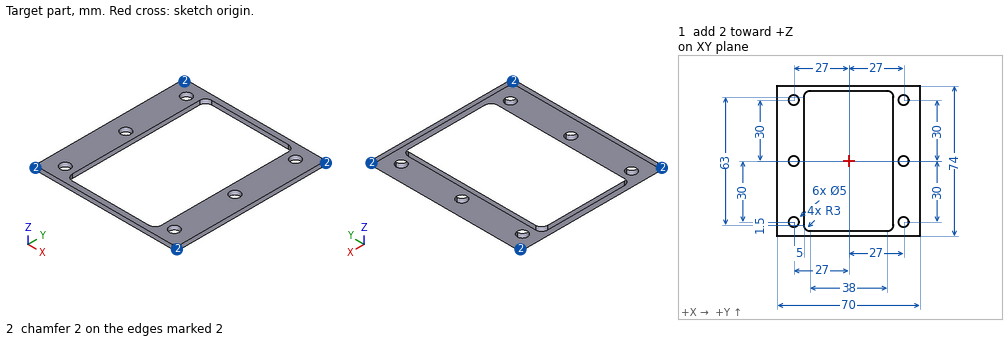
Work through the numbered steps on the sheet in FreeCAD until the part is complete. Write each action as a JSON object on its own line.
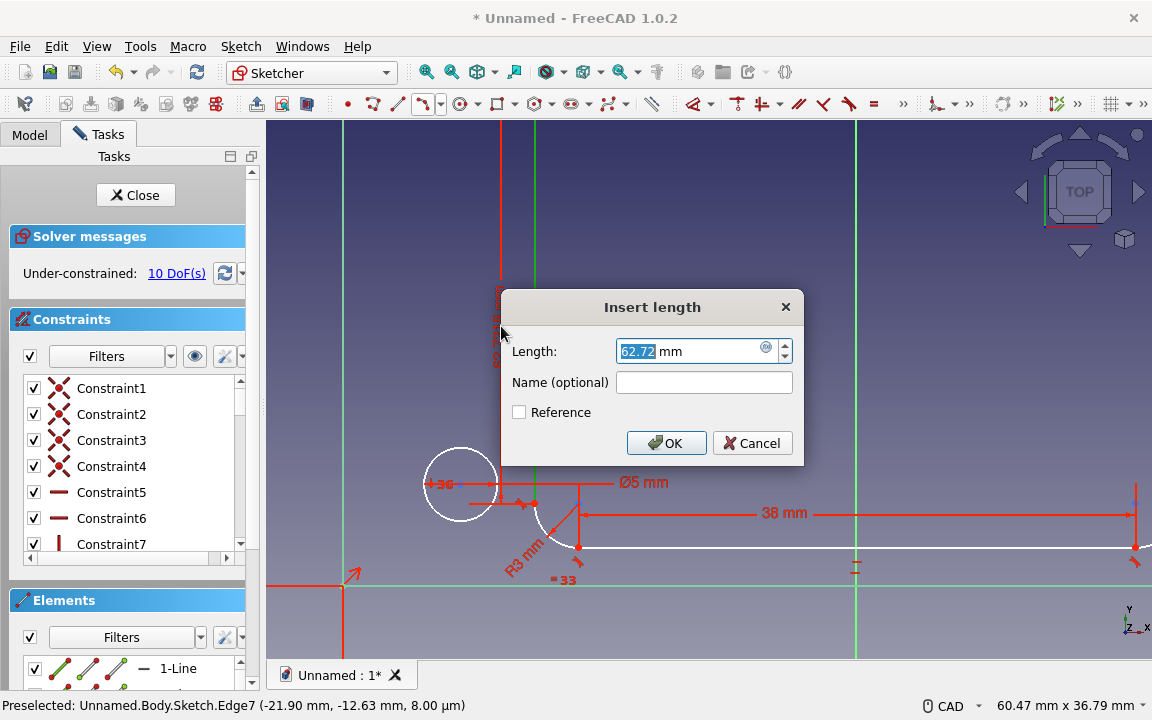
{"action": "type", "text": "63"}
{"action": "key", "text": "Return"}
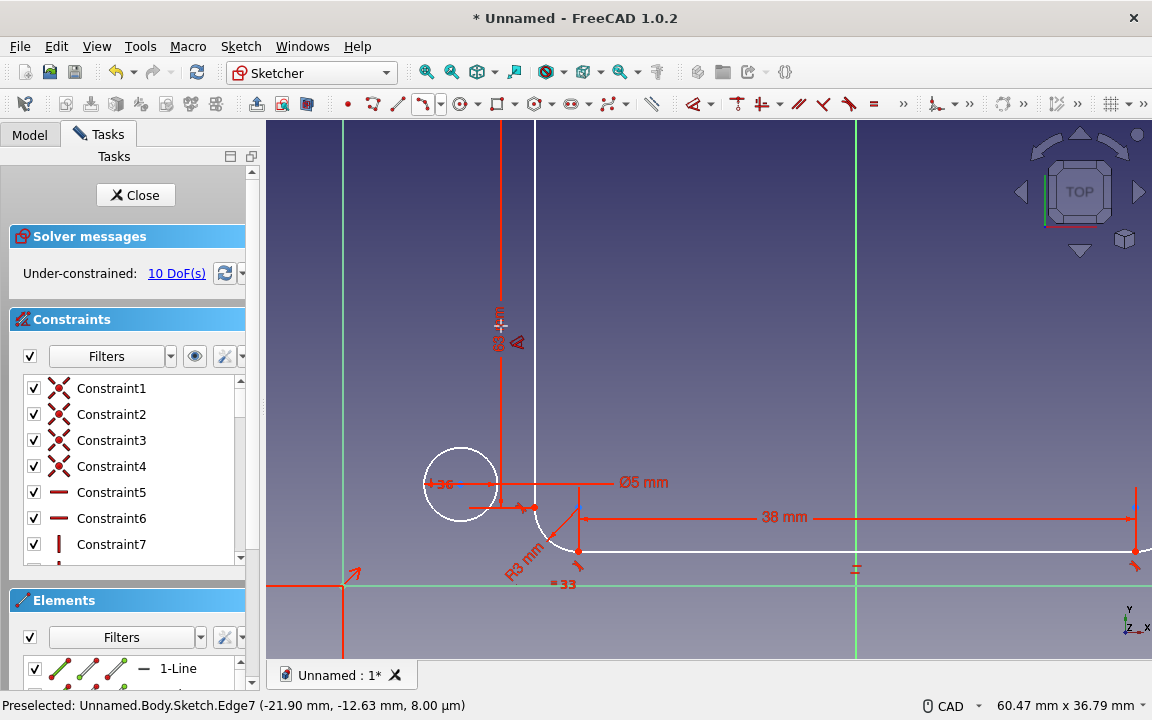
{"action": "left_click", "coordinate": [461, 484]}
{"action": "left_click", "coordinate": [658, 518]}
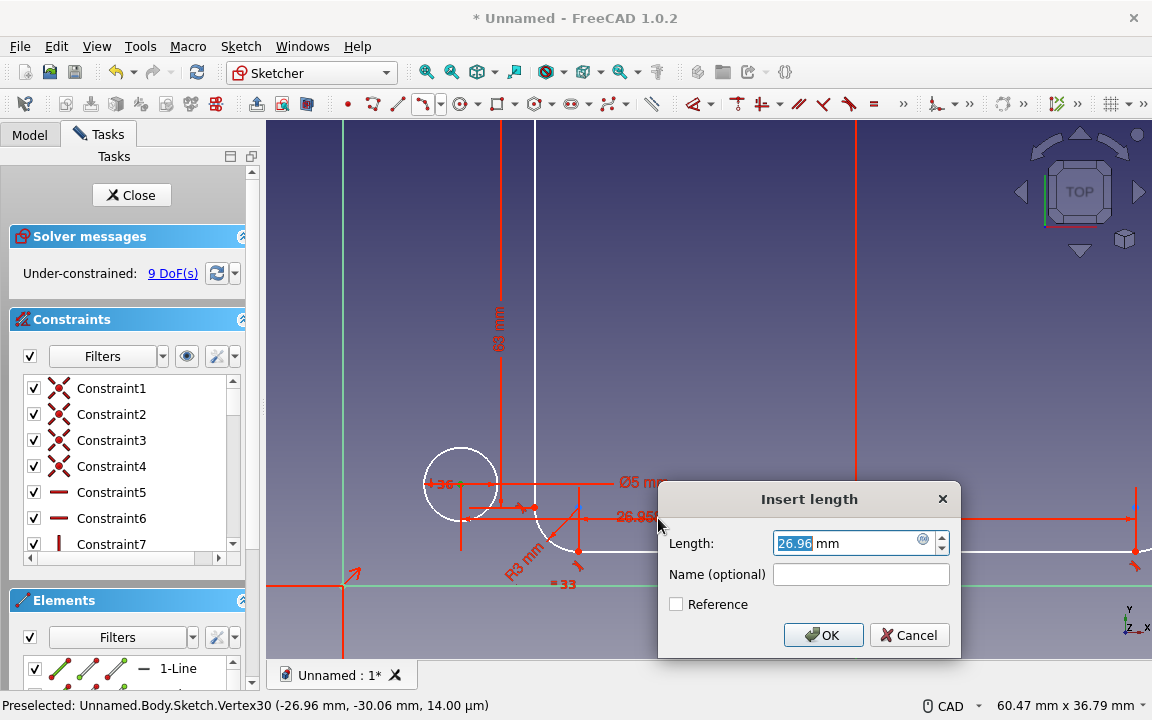
{"action": "type", "text": "27"}
{"action": "key", "text": "Return"}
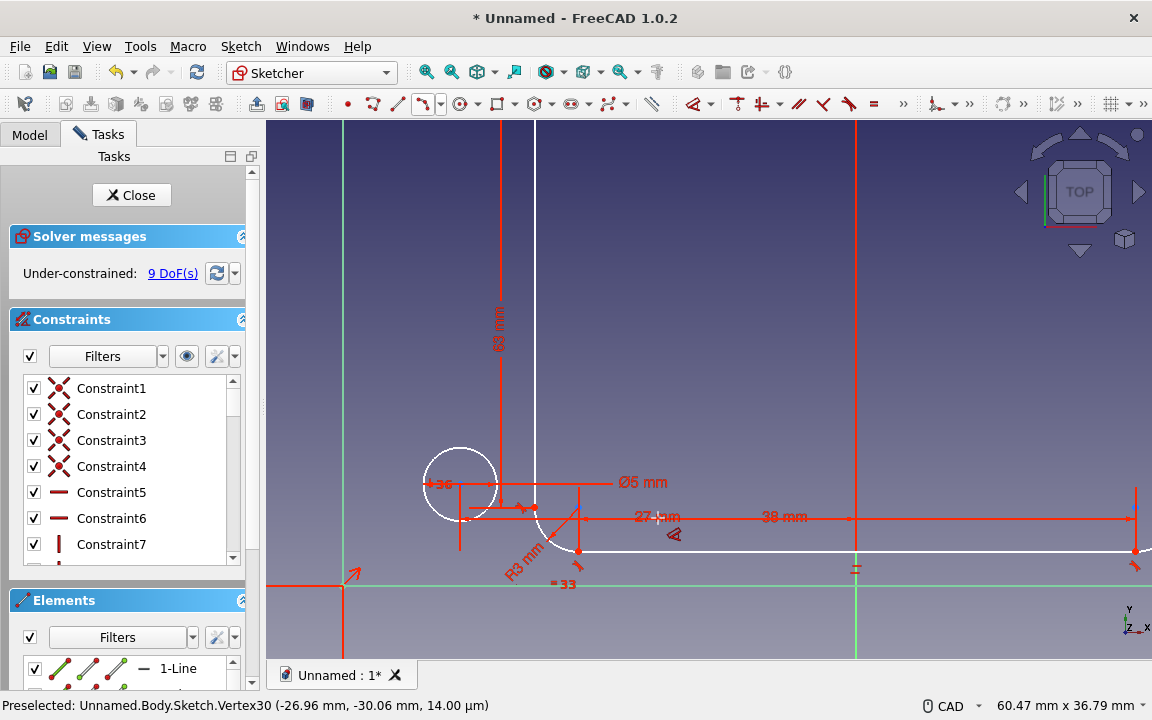
{"action": "left_click", "coordinate": [460, 484]}
{"action": "left_click", "coordinate": [426, 316]}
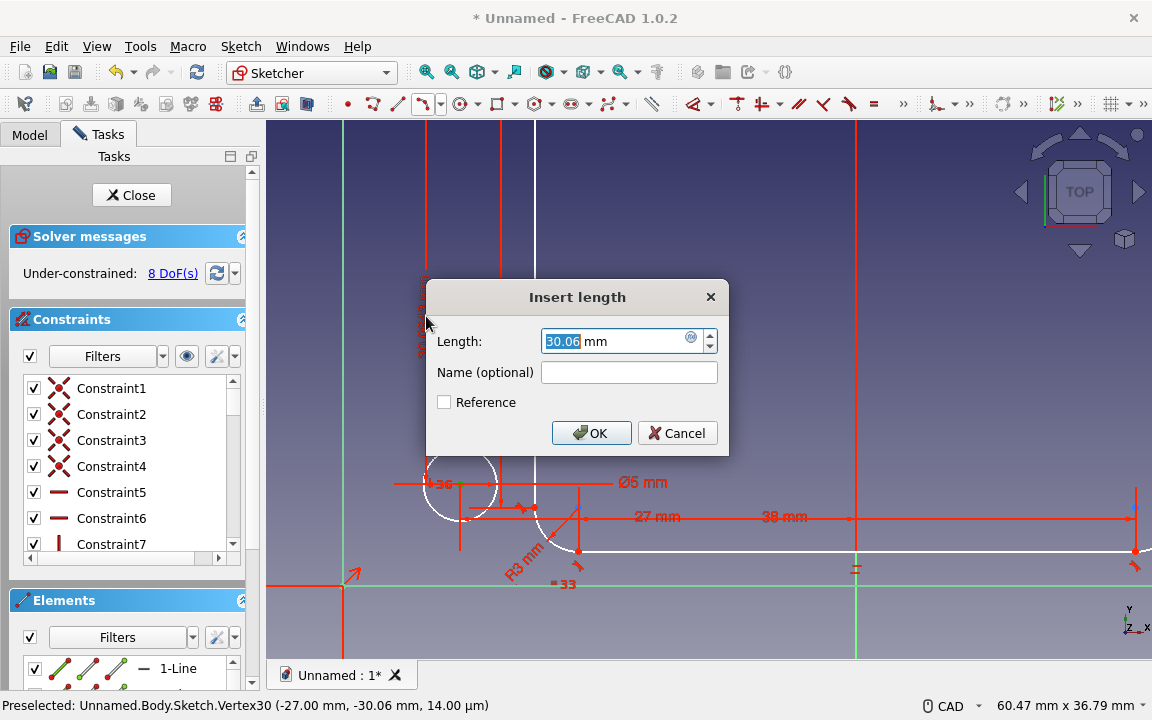
{"action": "type", "text": "30"}
{"action": "key", "text": "Return"}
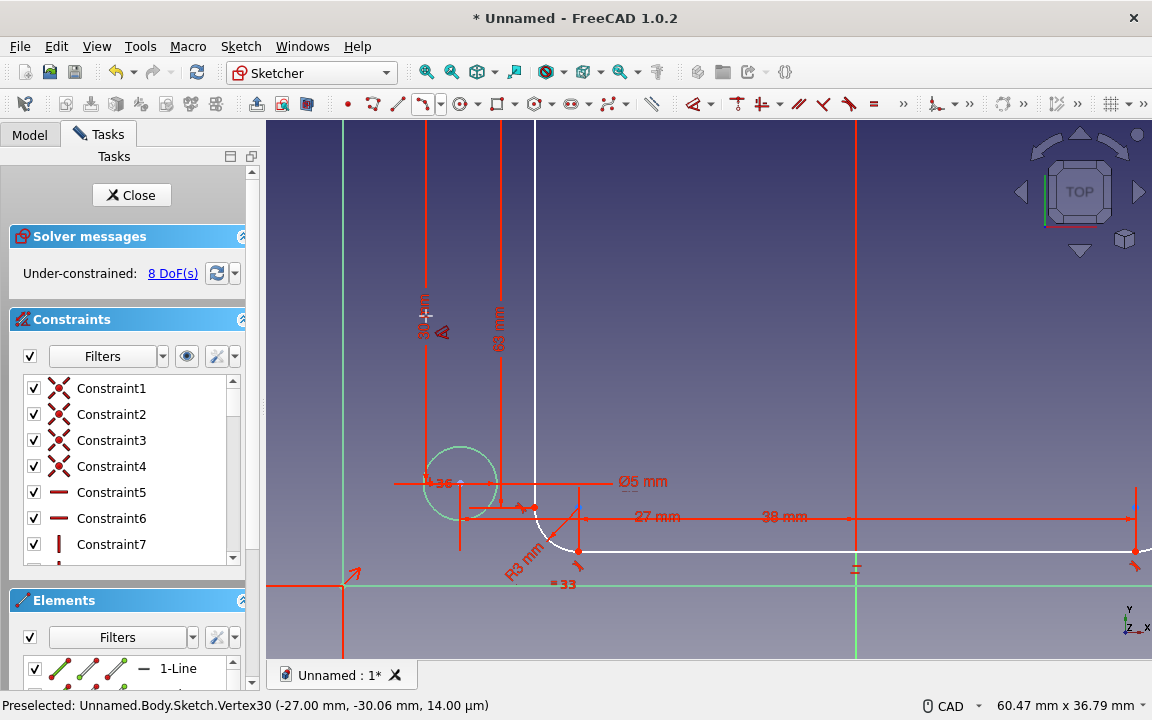
{"action": "scroll", "coordinate": [548, 538], "scroll_direction": "down", "scroll_amount": 6}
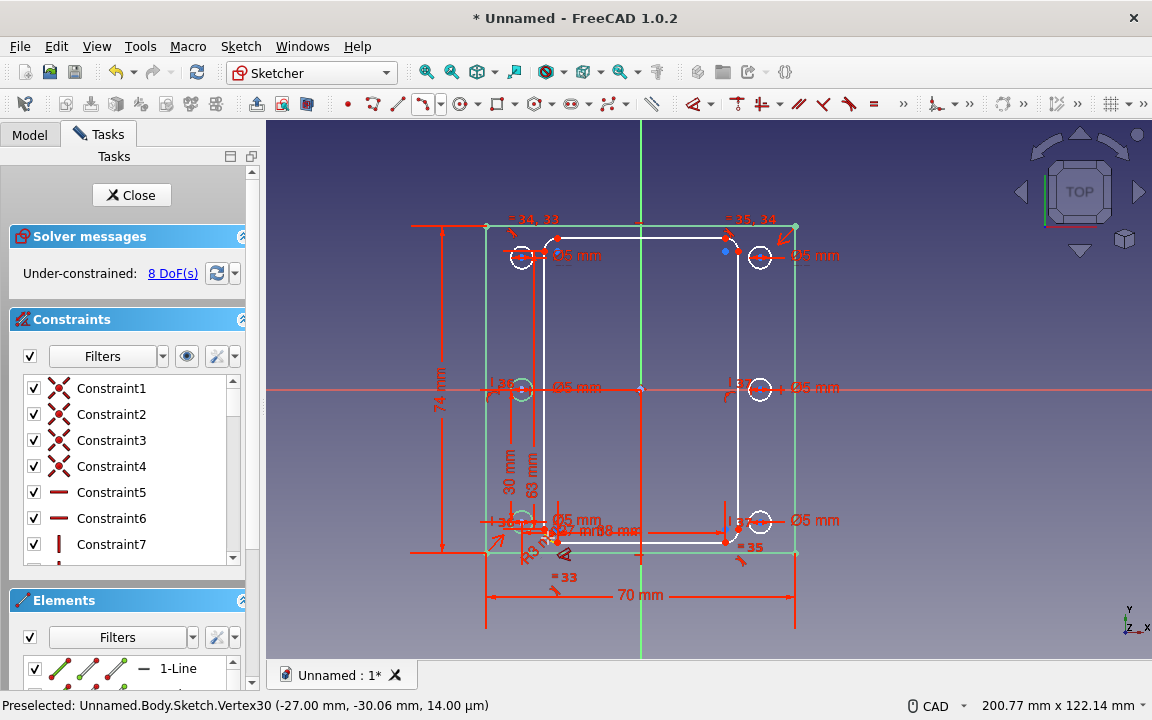
{"action": "left_click", "coordinate": [760, 522]}
{"action": "left_click", "coordinate": [701, 356]}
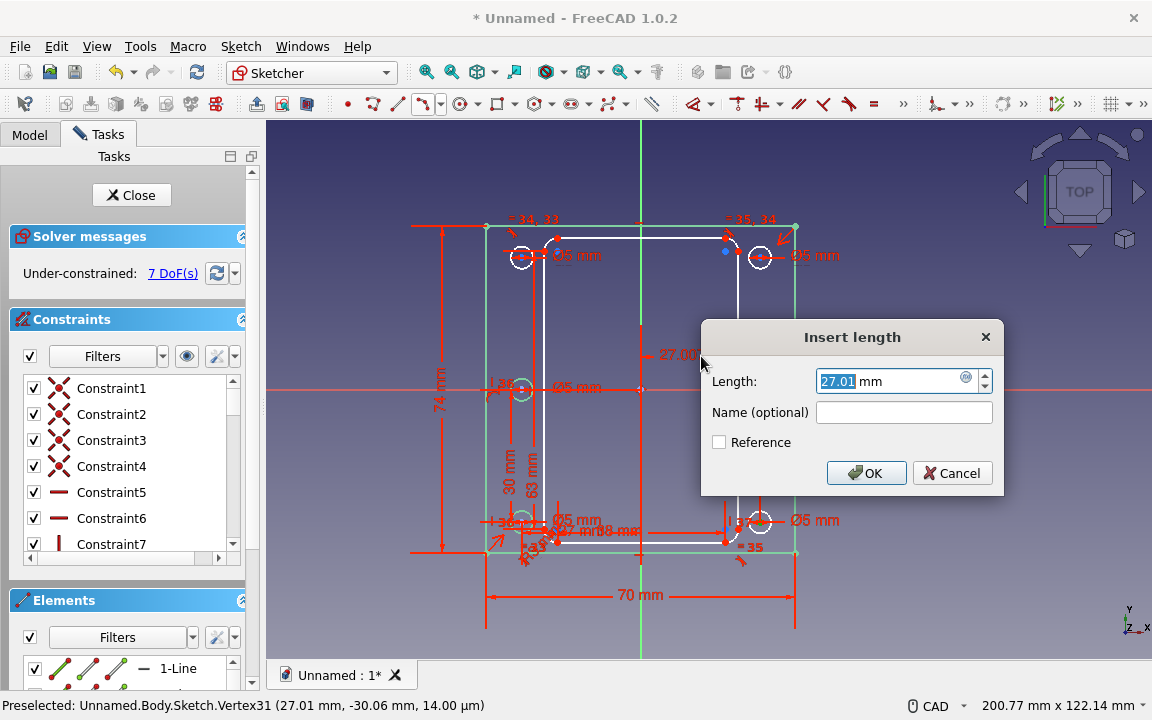
{"action": "type", "text": "27"}
{"action": "key", "text": "Return"}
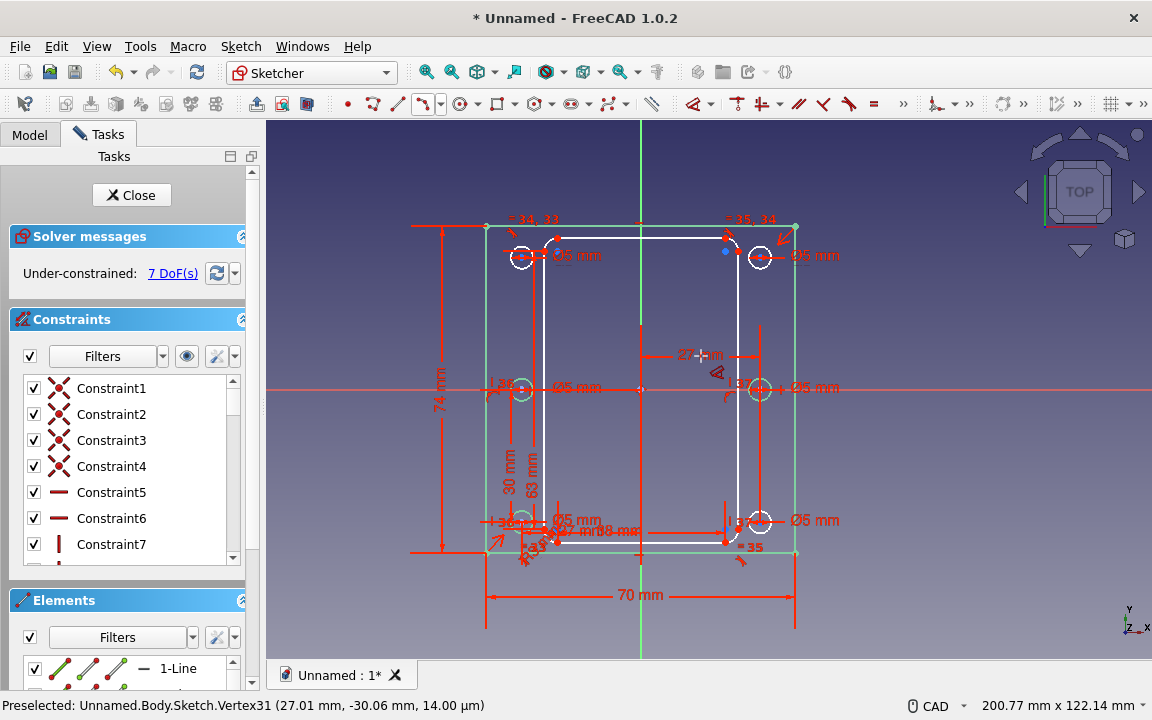
{"action": "left_click", "coordinate": [760, 522]}
{"action": "left_click", "coordinate": [607, 456]}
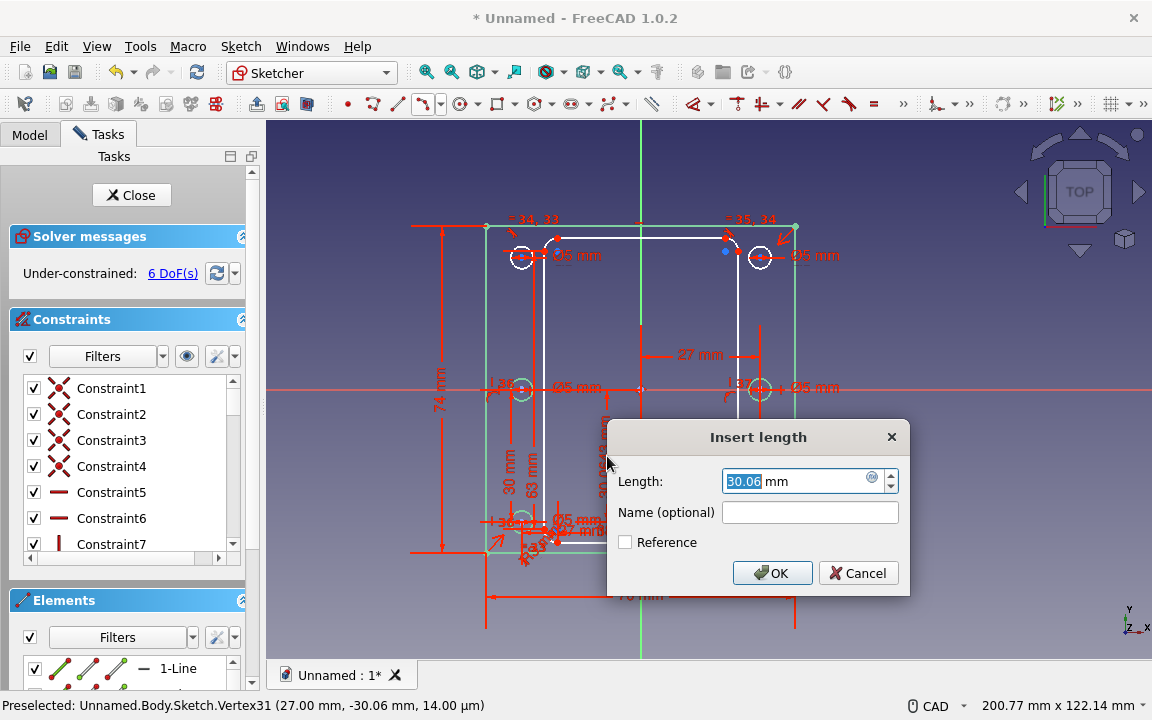
{"action": "type", "text": "30"}
{"action": "key", "text": "Return"}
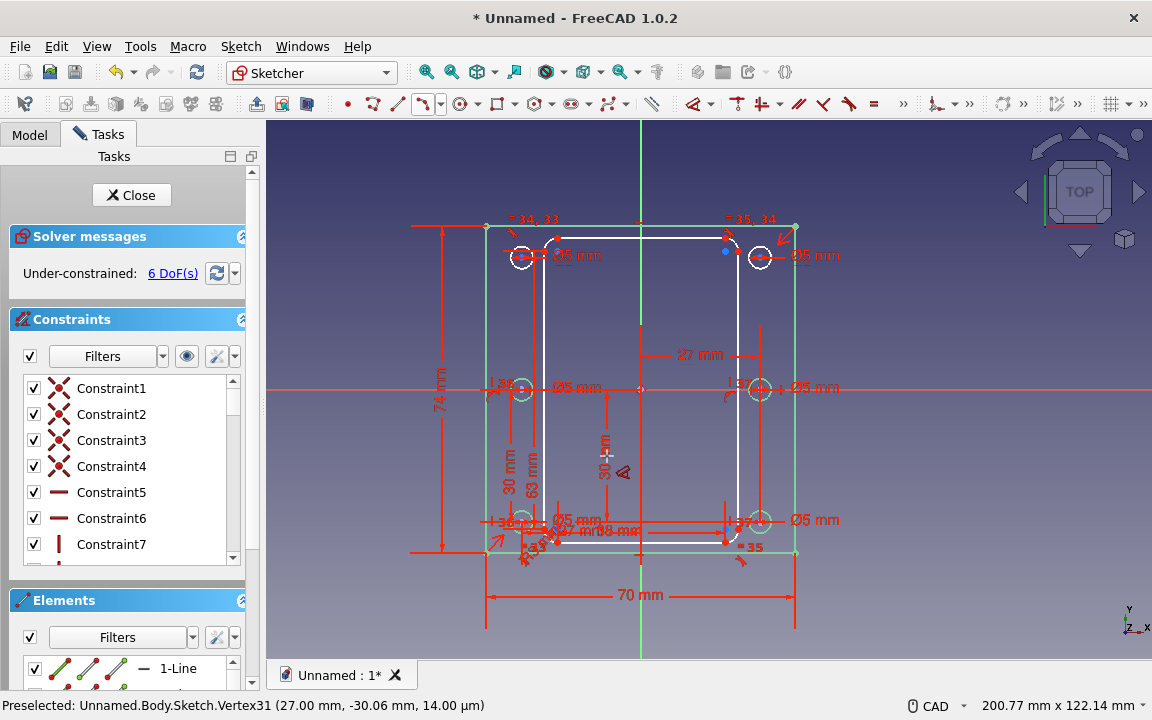
{"action": "left_click", "coordinate": [522, 258]}
{"action": "left_click", "coordinate": [581, 424]}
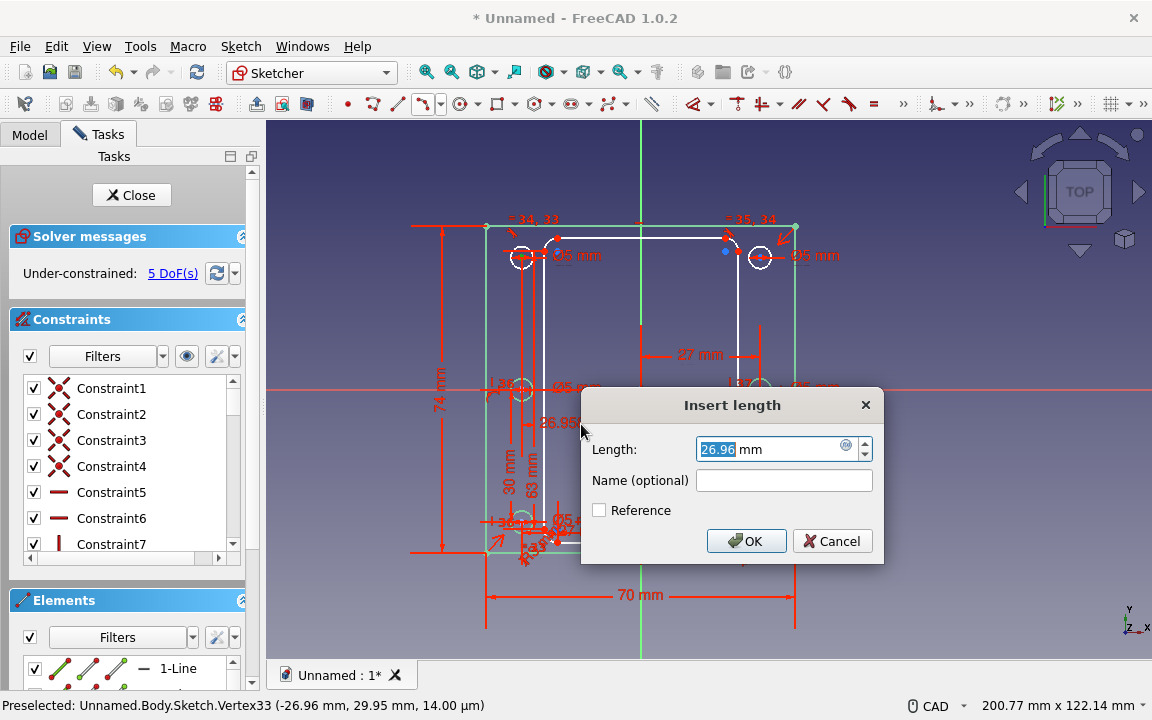
{"action": "type", "text": "27"}
{"action": "key", "text": "Return"}